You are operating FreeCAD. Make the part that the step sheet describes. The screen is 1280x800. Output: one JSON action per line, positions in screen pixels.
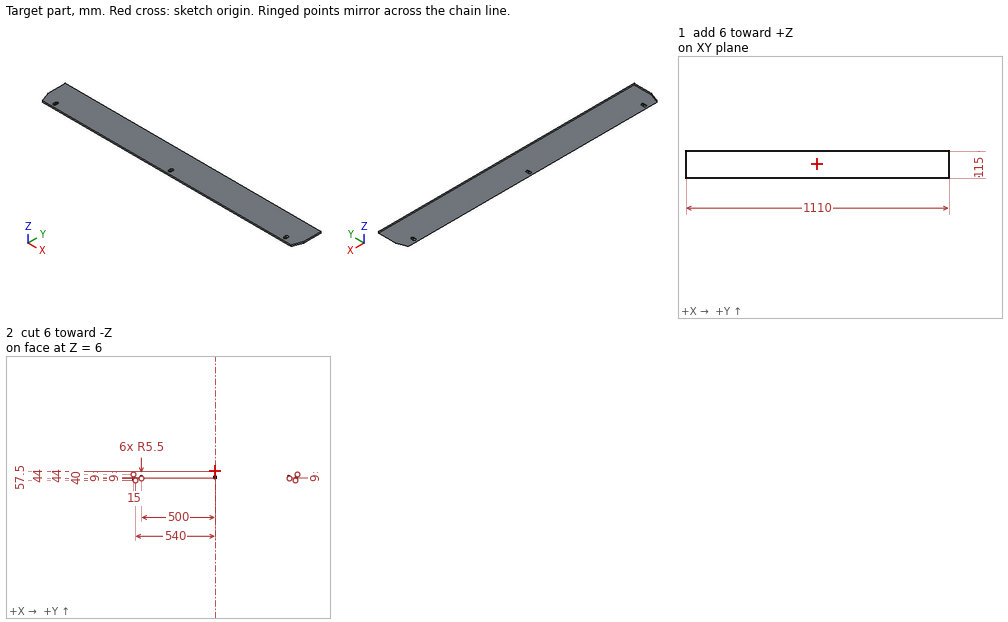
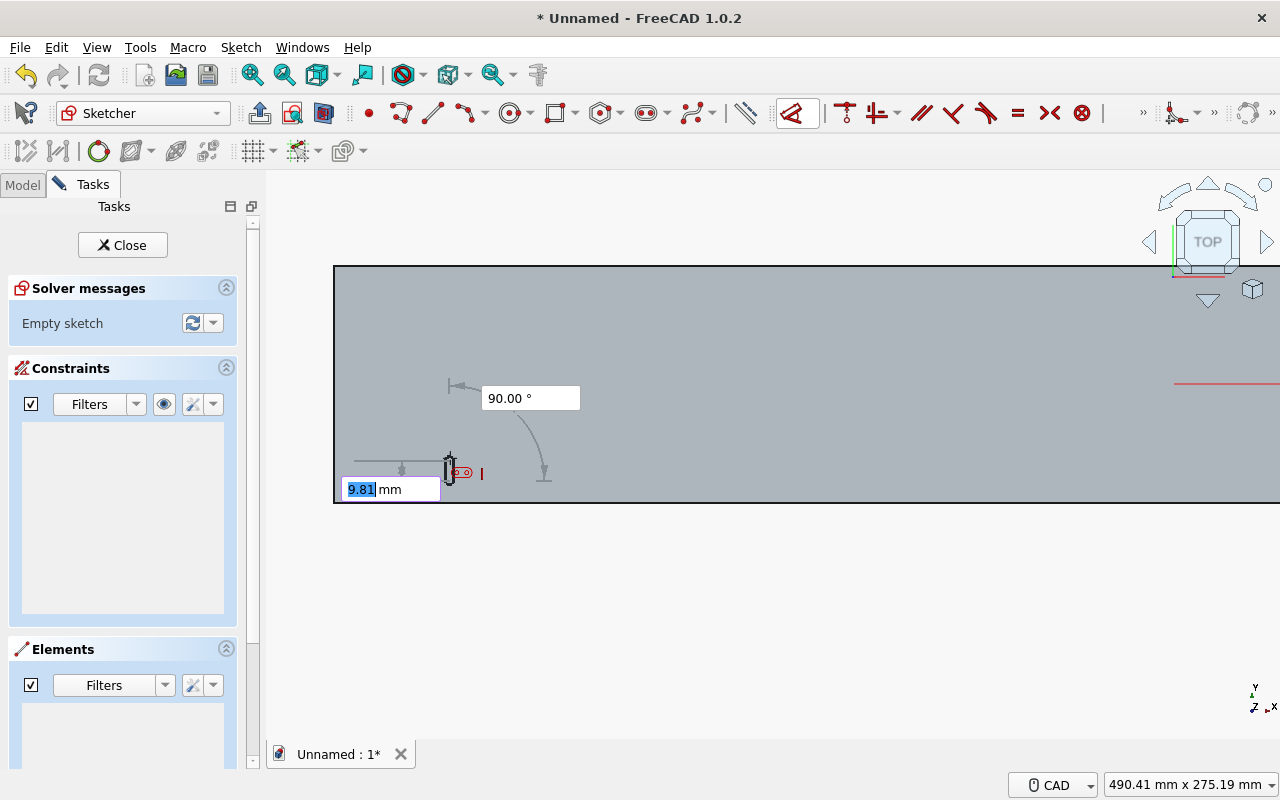
{"action": "left_click", "coordinate": [449, 457]}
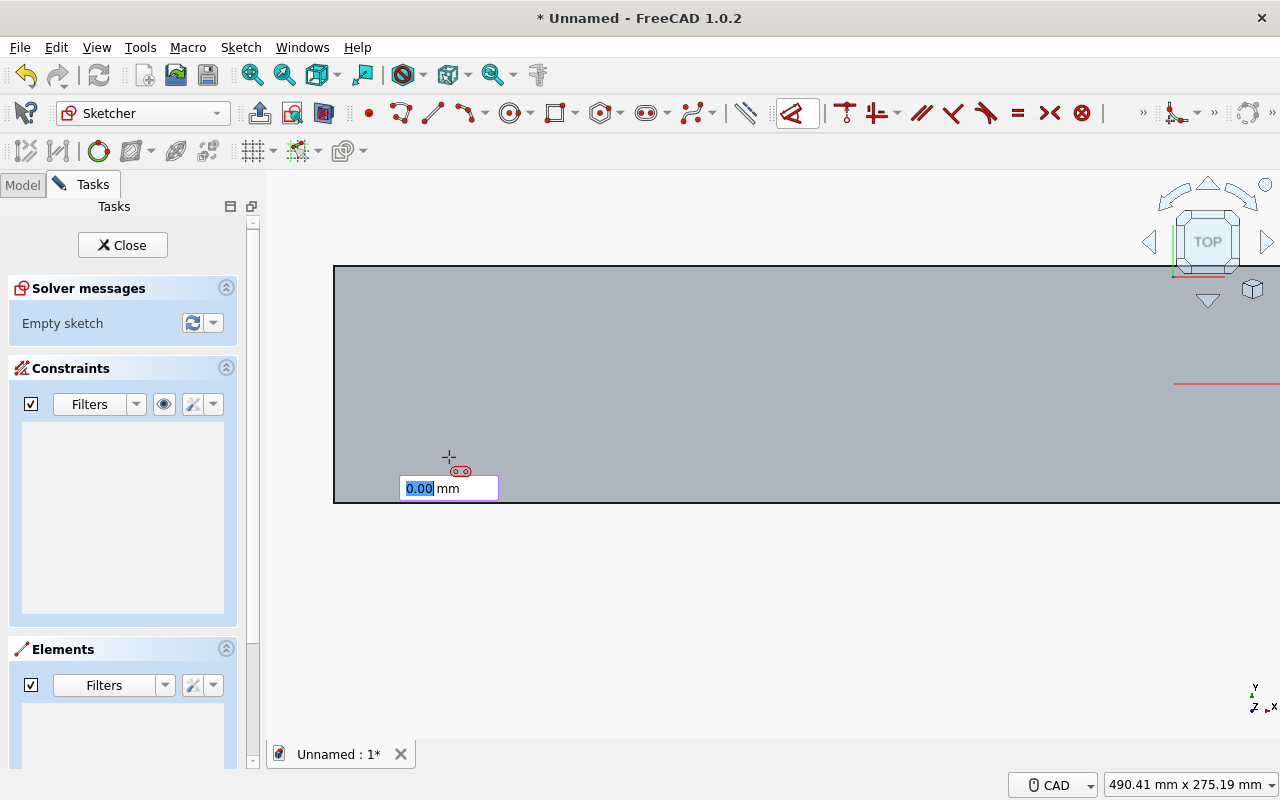
{"action": "scroll", "coordinate": [459, 466], "scroll_direction": "up", "scroll_amount": 2}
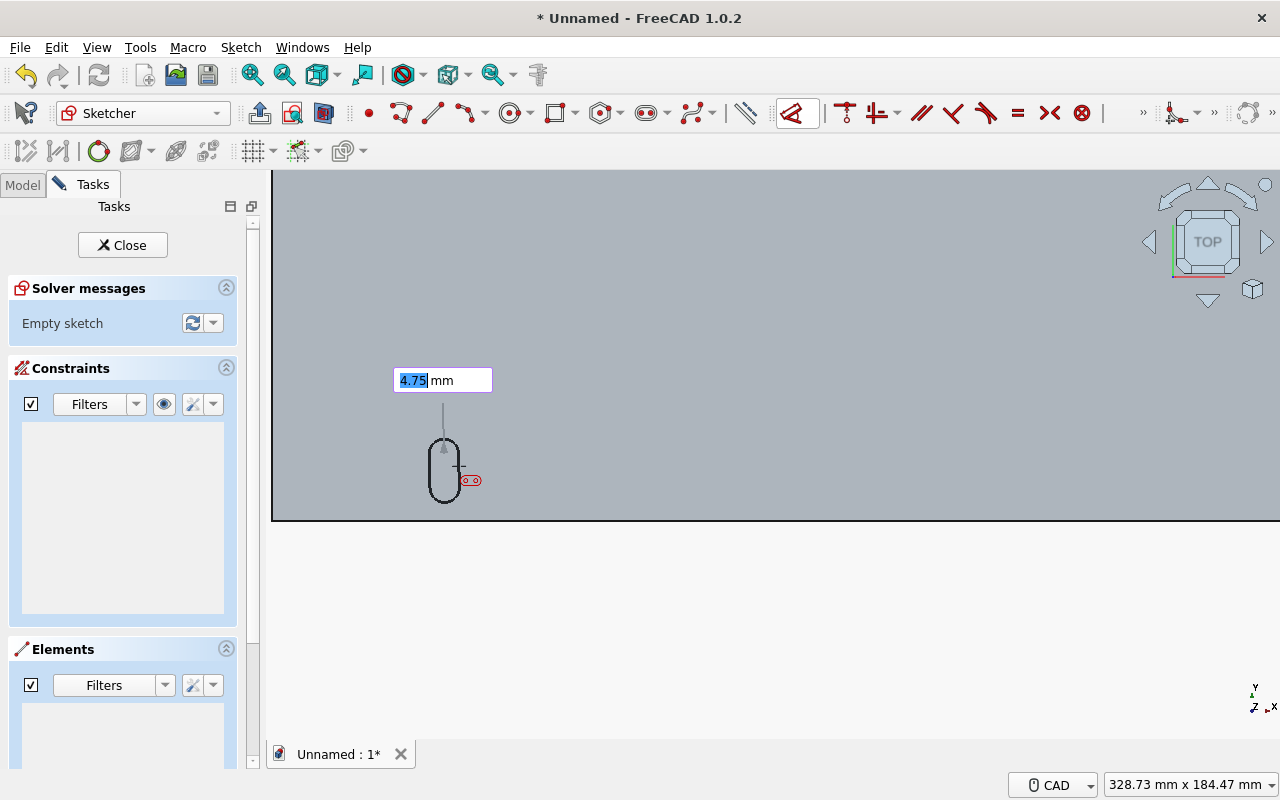
{"action": "left_click", "coordinate": [459, 466]}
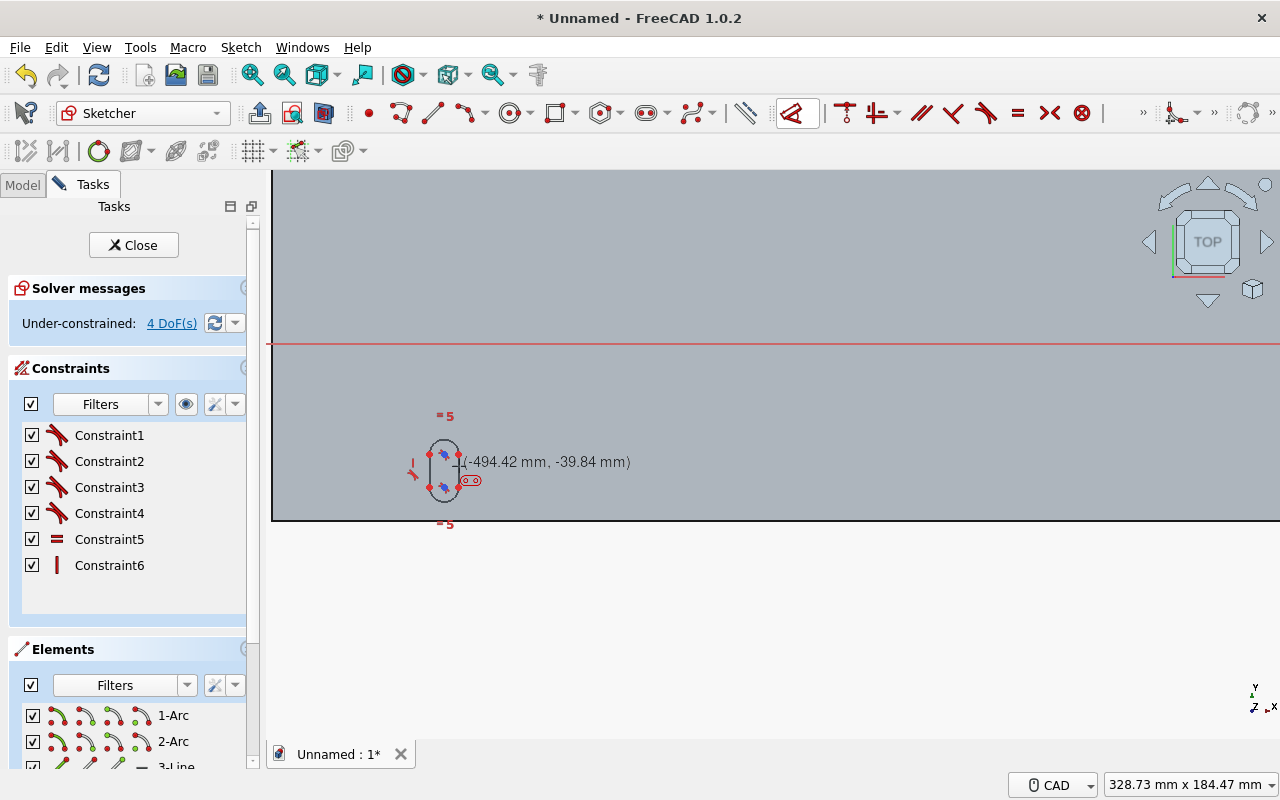
{"action": "scroll", "coordinate": [451, 459], "scroll_direction": "down", "scroll_amount": 9}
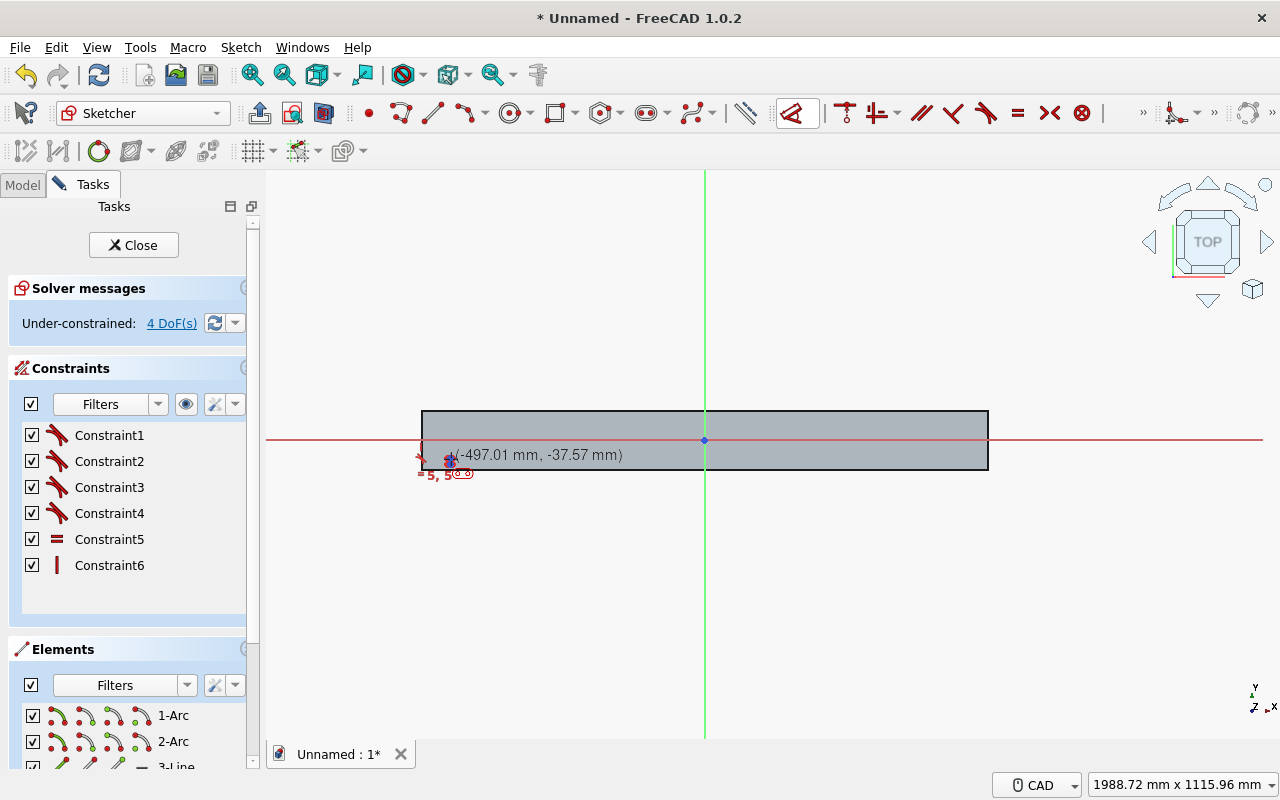
{"action": "scroll", "coordinate": [705, 463], "scroll_direction": "up", "scroll_amount": 11}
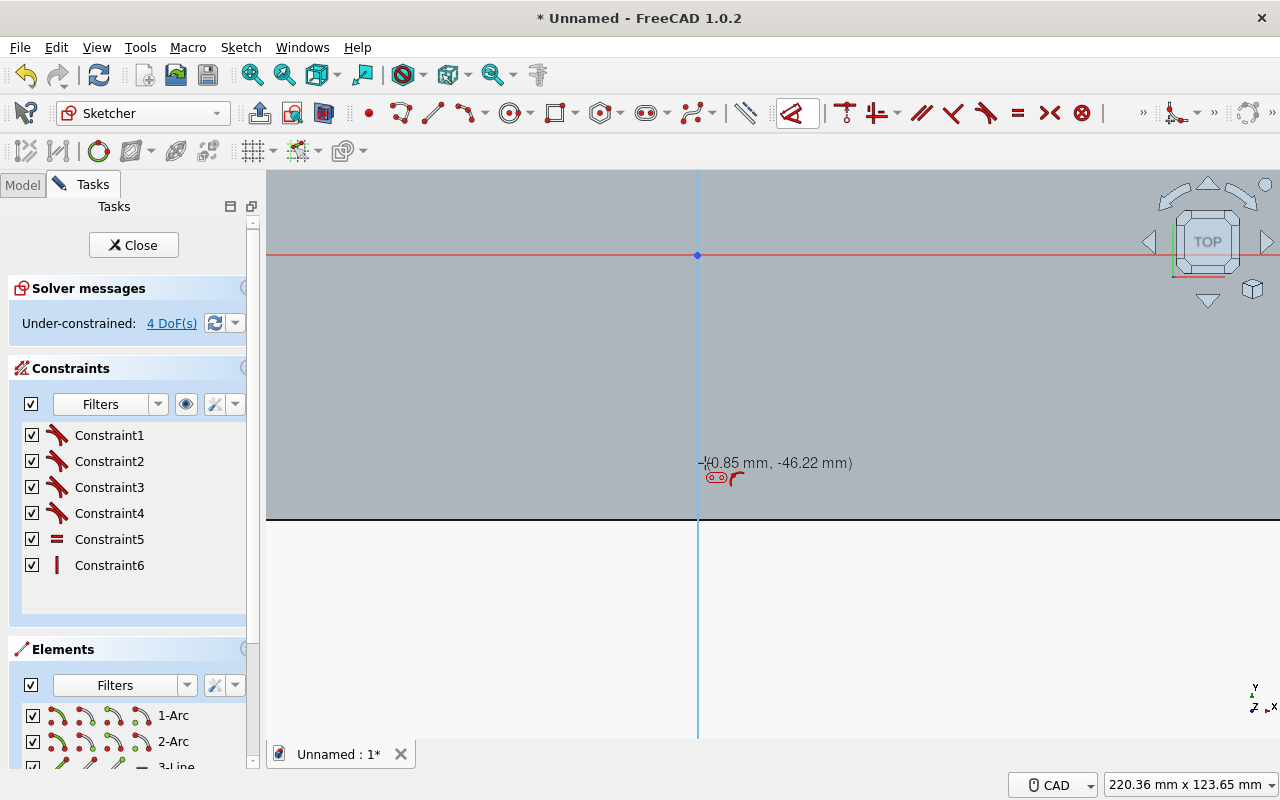
{"action": "scroll", "coordinate": [705, 463], "scroll_direction": "down", "scroll_amount": 11}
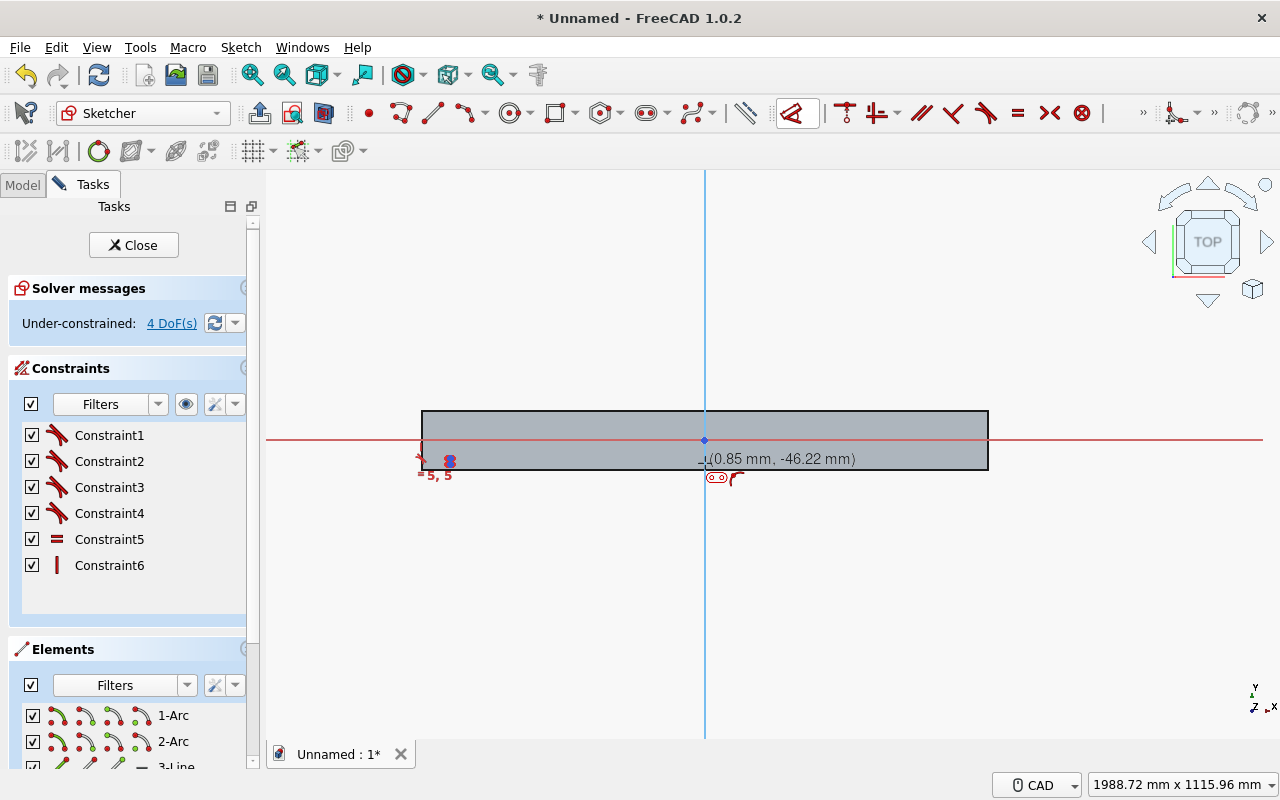
{"action": "left_click", "coordinate": [705, 463]}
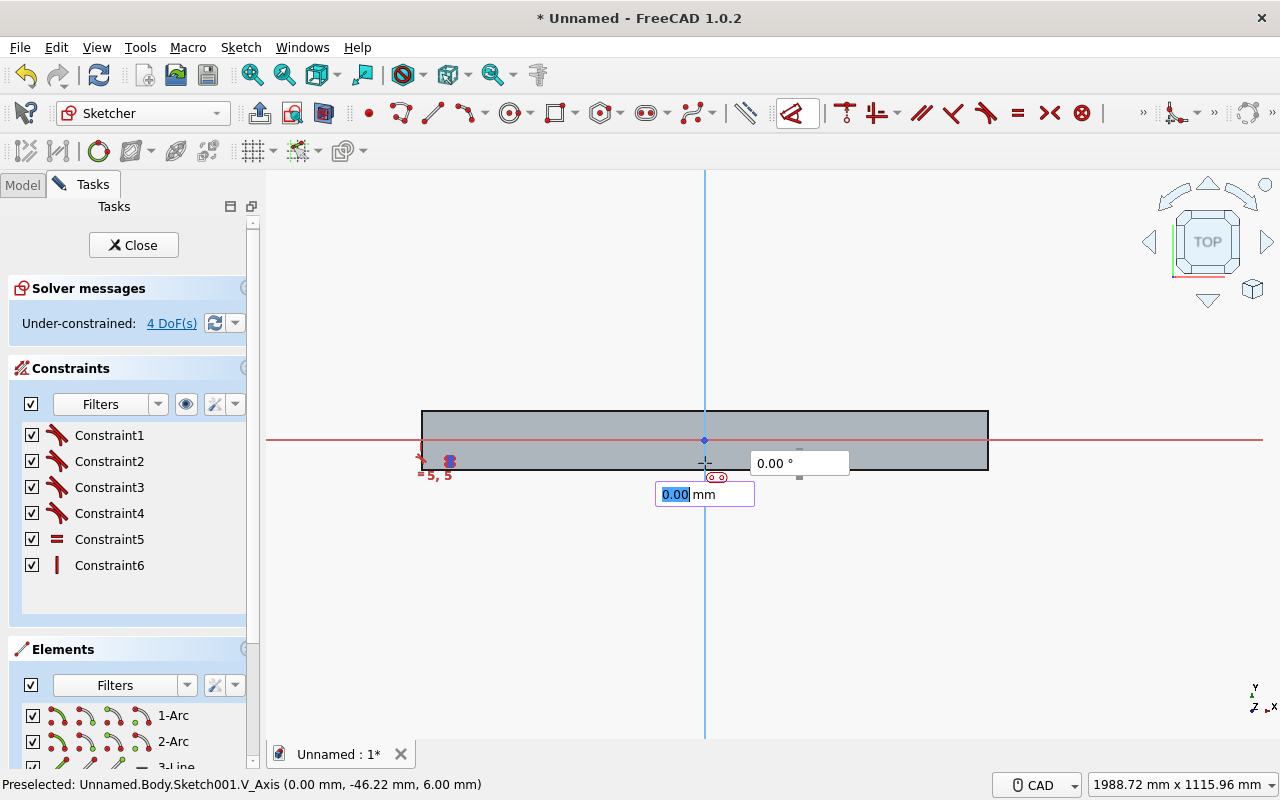
{"action": "scroll", "coordinate": [705, 458], "scroll_direction": "up", "scroll_amount": 7}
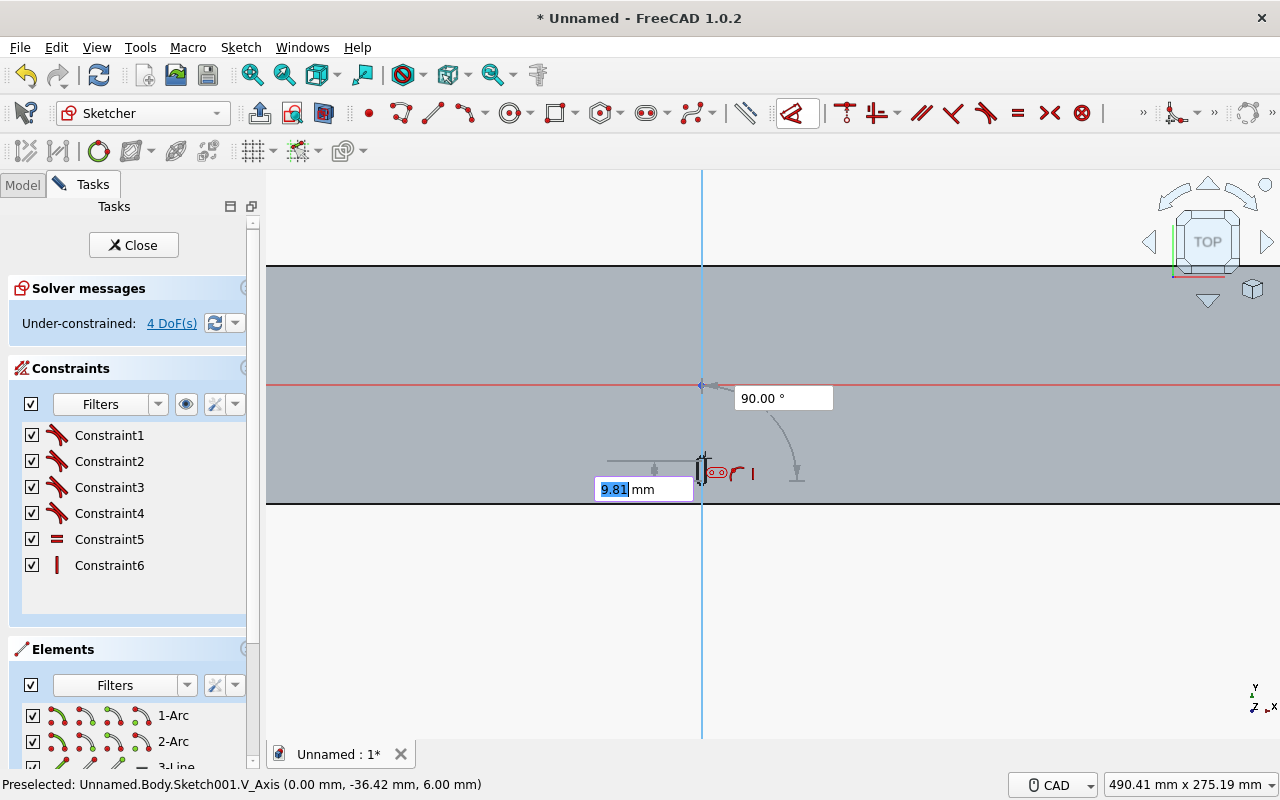
{"action": "left_click", "coordinate": [711, 458]}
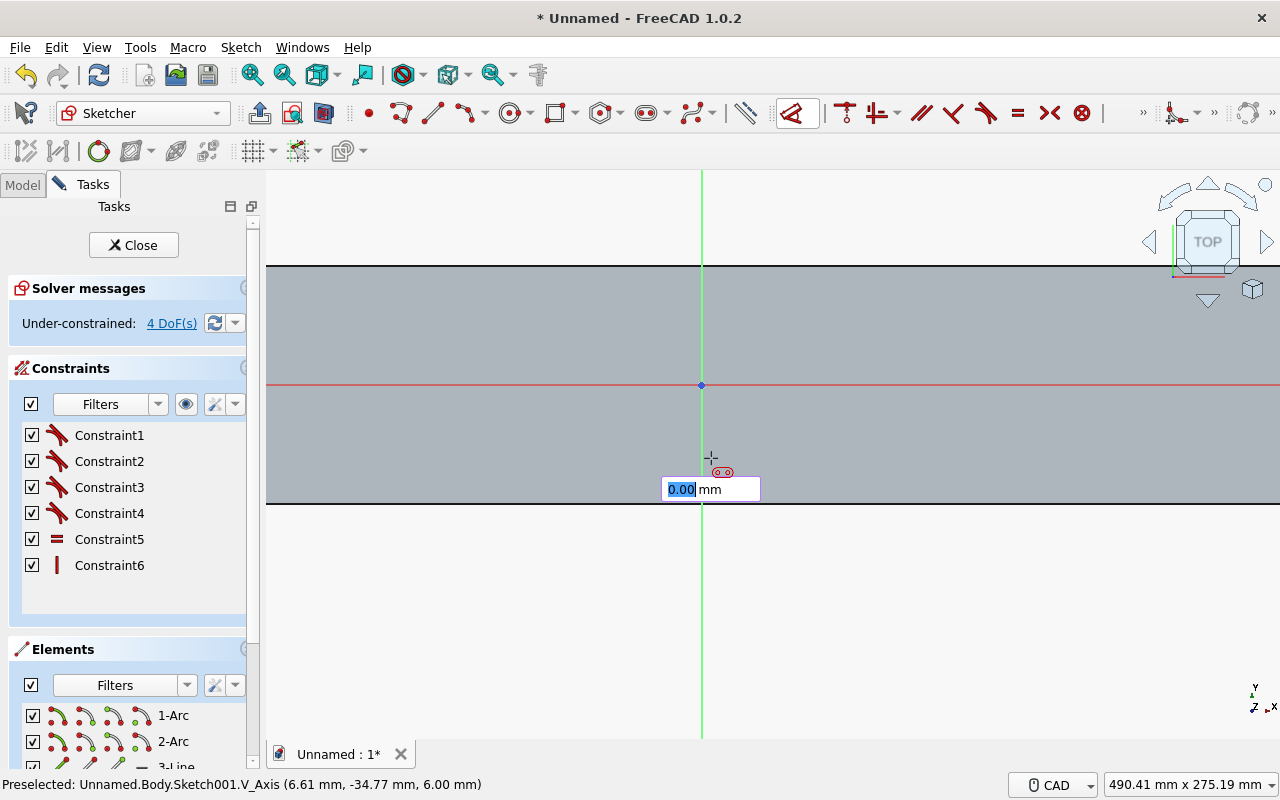
{"action": "scroll", "coordinate": [713, 467], "scroll_direction": "up", "scroll_amount": 2}